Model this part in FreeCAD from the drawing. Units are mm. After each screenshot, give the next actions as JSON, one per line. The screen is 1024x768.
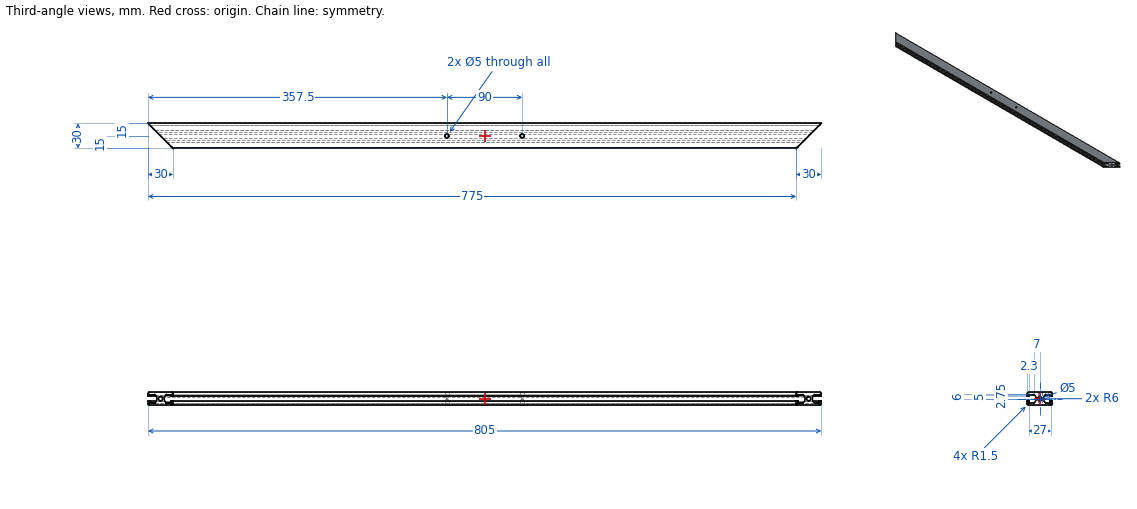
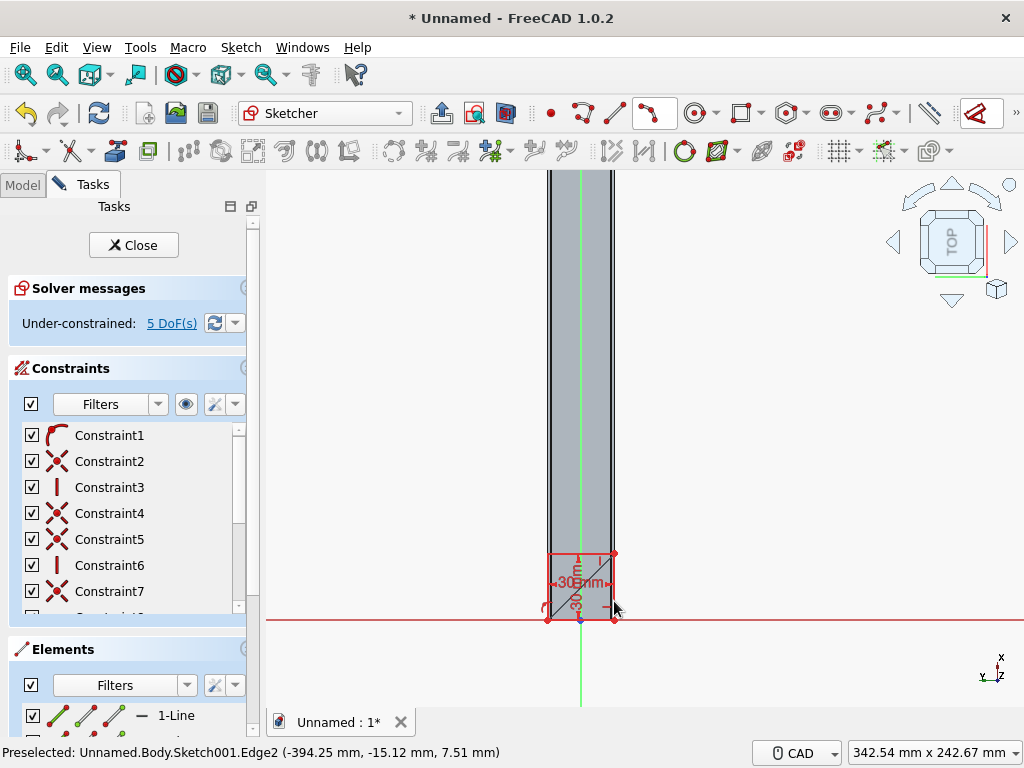
{"action": "scroll", "coordinate": [575, 618], "scroll_direction": "down", "scroll_amount": 8}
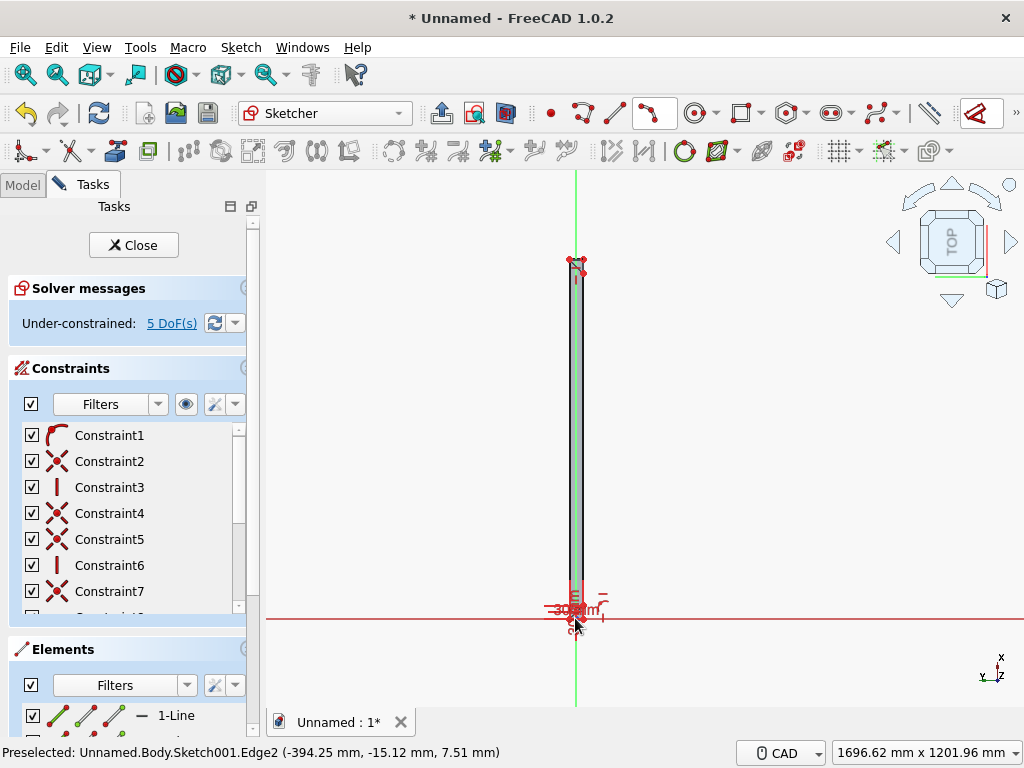
{"action": "scroll", "coordinate": [583, 269], "scroll_direction": "up", "scroll_amount": 8}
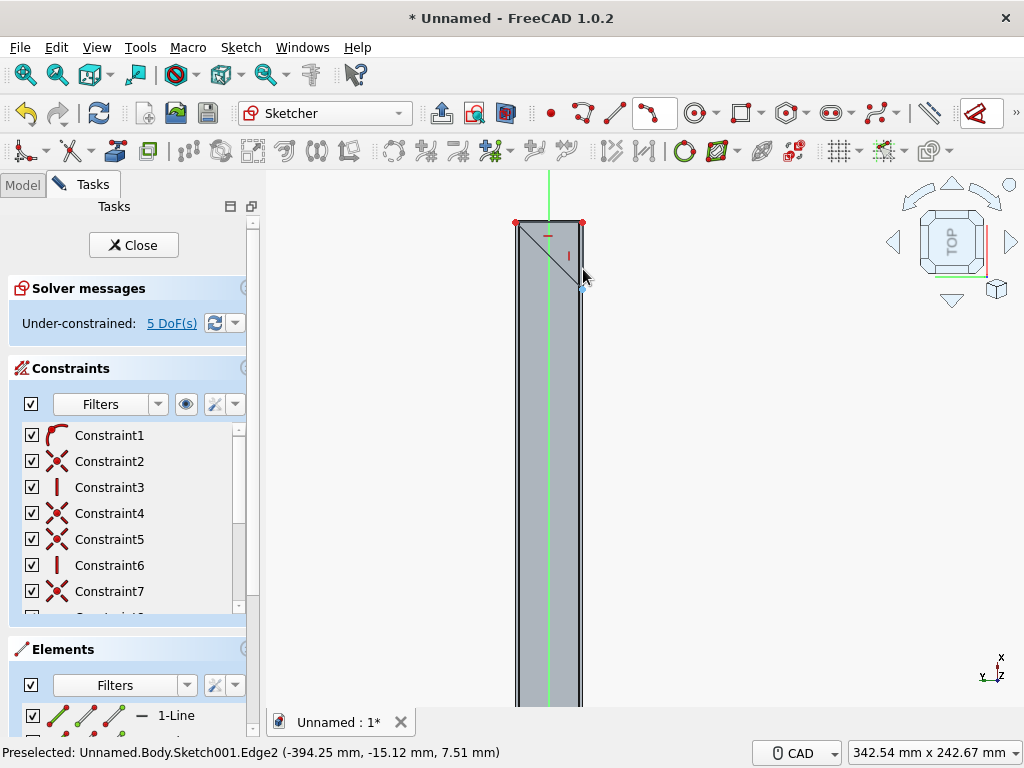
{"action": "left_click", "coordinate": [583, 269]}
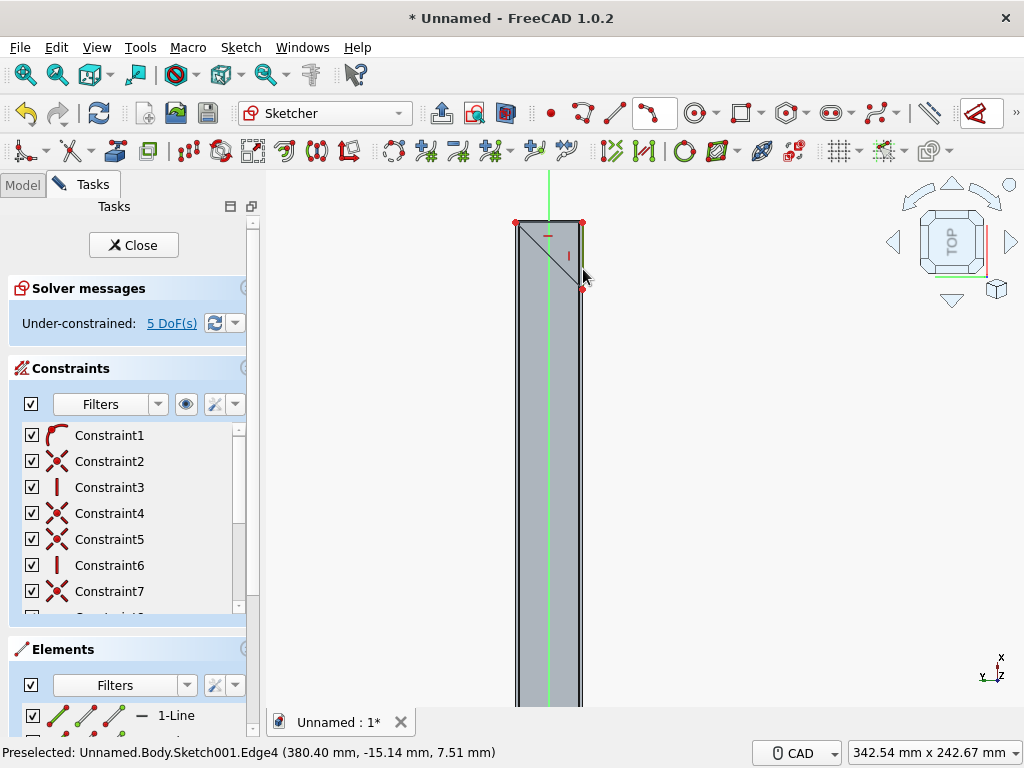
{"action": "left_click", "coordinate": [998, 114]}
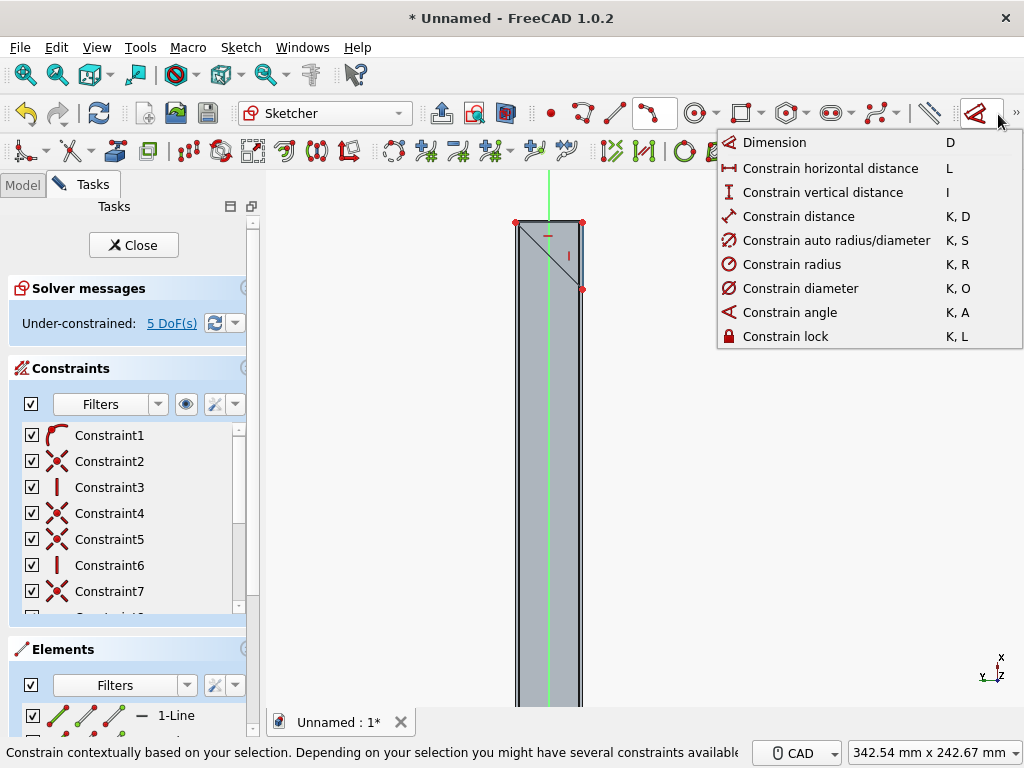
{"action": "left_click", "coordinate": [870, 192]}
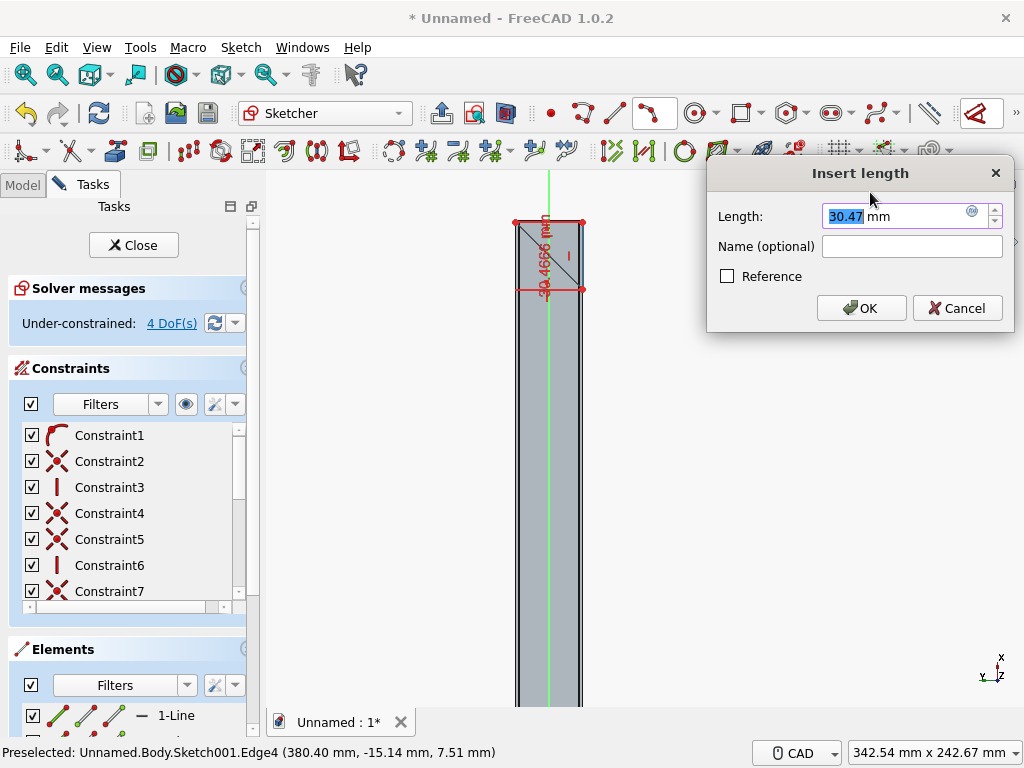
{"action": "type", "text": "30"}
{"action": "key", "text": "Return"}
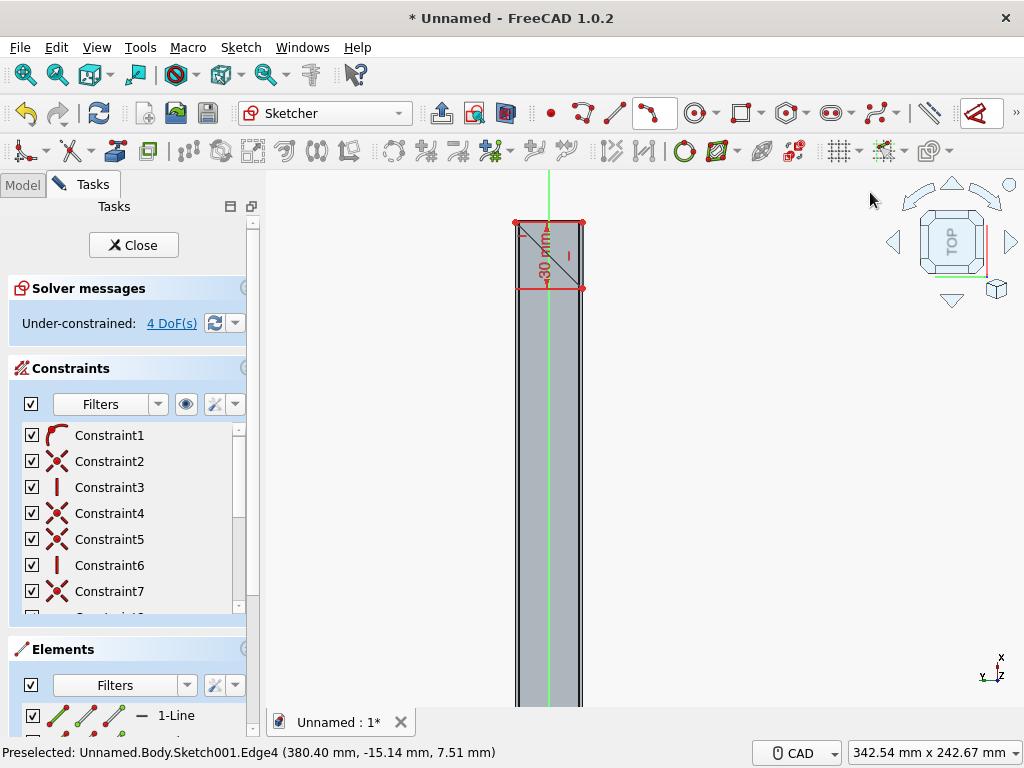
{"action": "left_click", "coordinate": [562, 222]}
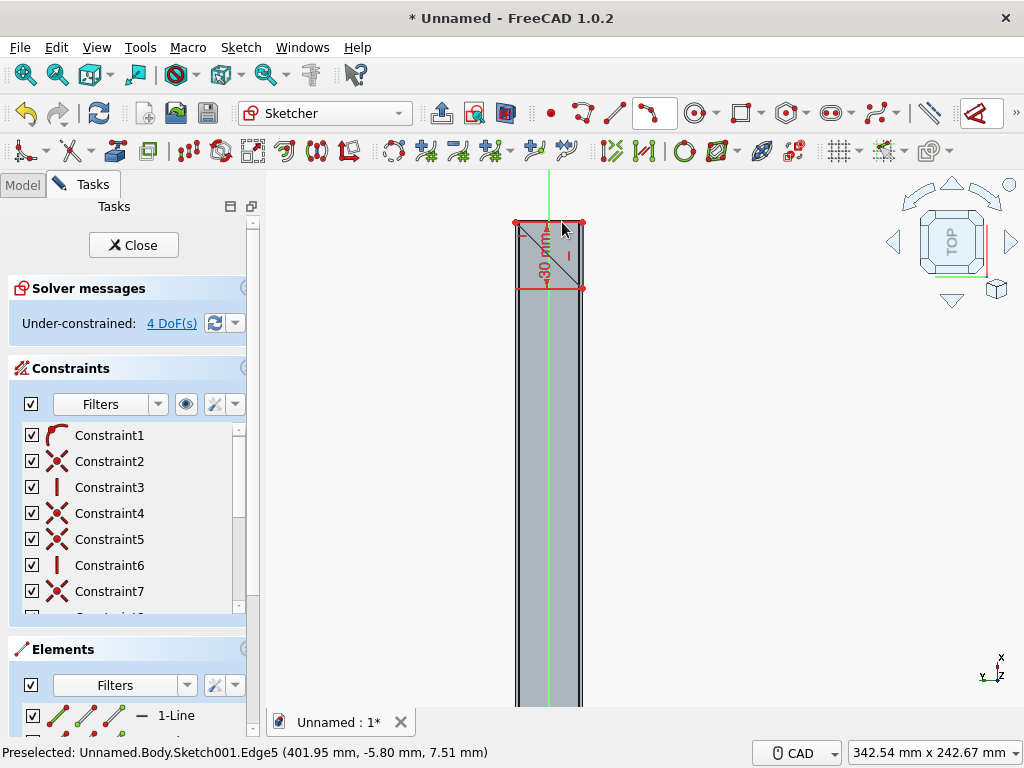
{"action": "left_click", "coordinate": [998, 114]}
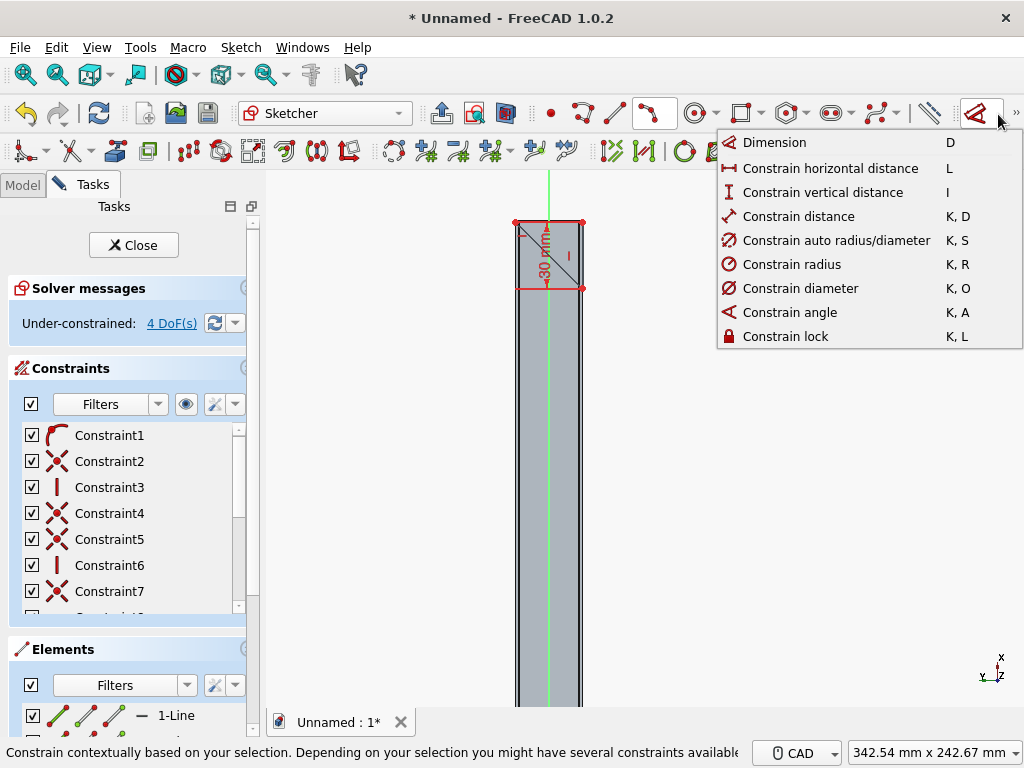
{"action": "left_click", "coordinate": [870, 168]}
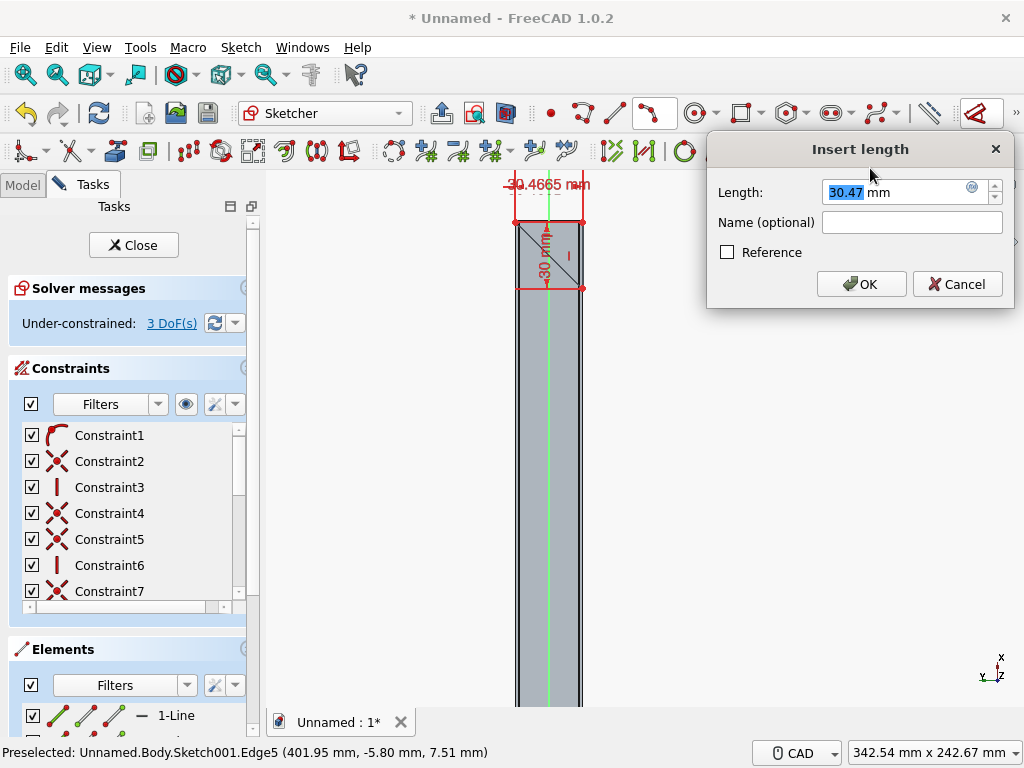
{"action": "type", "text": "30"}
{"action": "key", "text": "Return"}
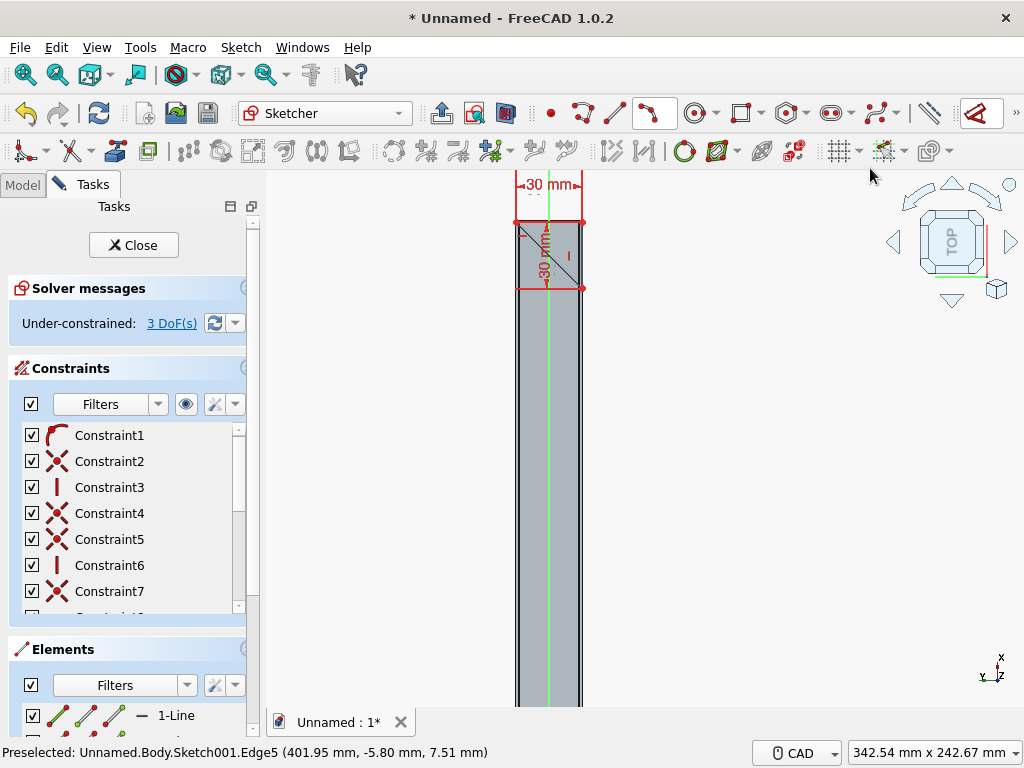
{"action": "scroll", "coordinate": [583, 268], "scroll_direction": "down", "scroll_amount": 8}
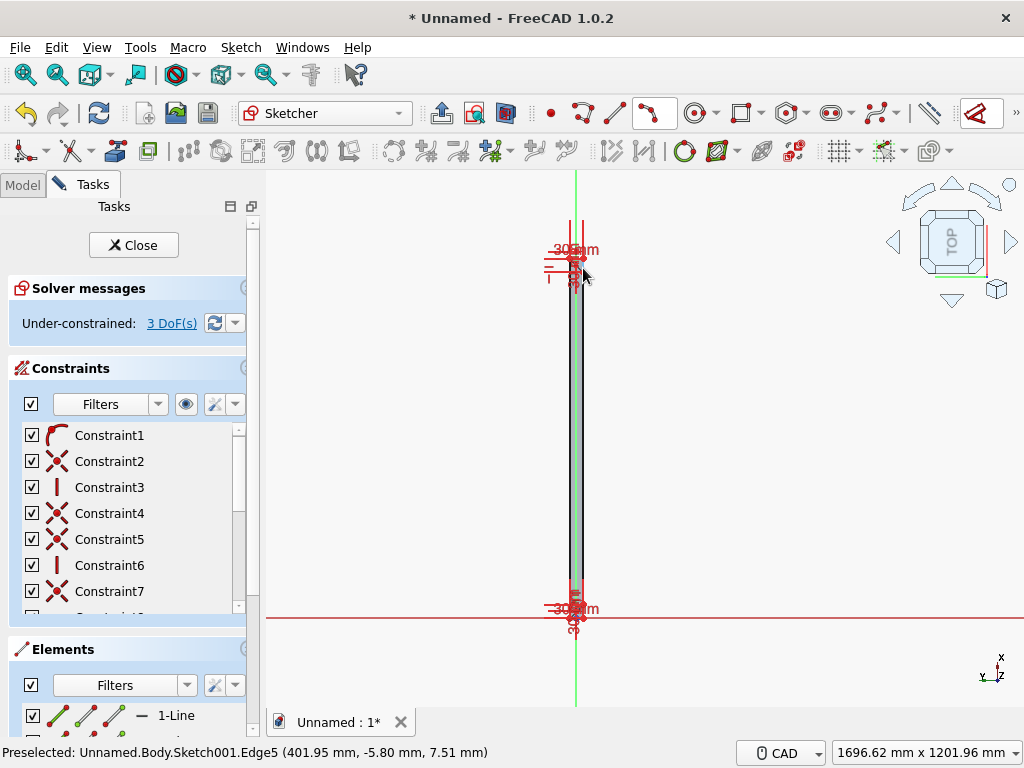
{"action": "scroll", "coordinate": [570, 618], "scroll_direction": "up", "scroll_amount": 9}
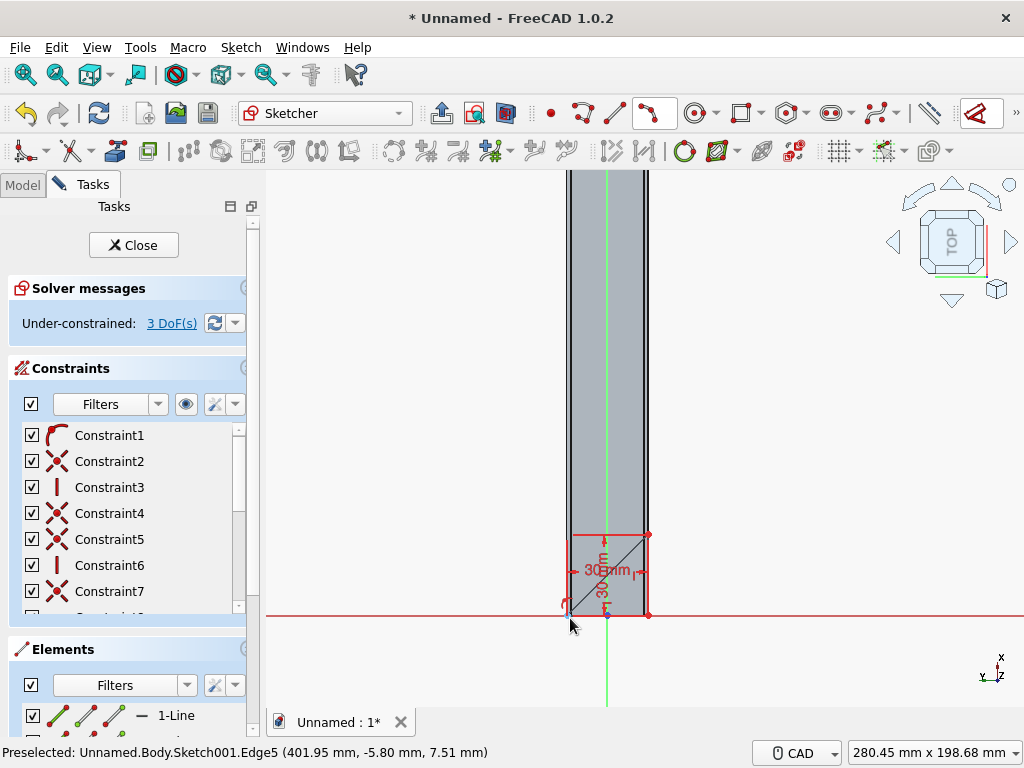
{"action": "left_click", "coordinate": [567, 616]}